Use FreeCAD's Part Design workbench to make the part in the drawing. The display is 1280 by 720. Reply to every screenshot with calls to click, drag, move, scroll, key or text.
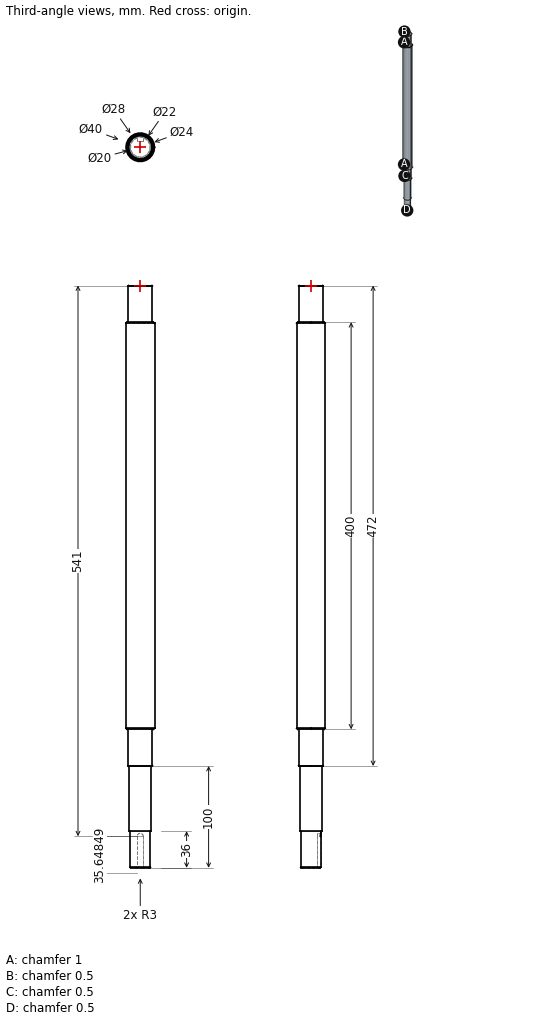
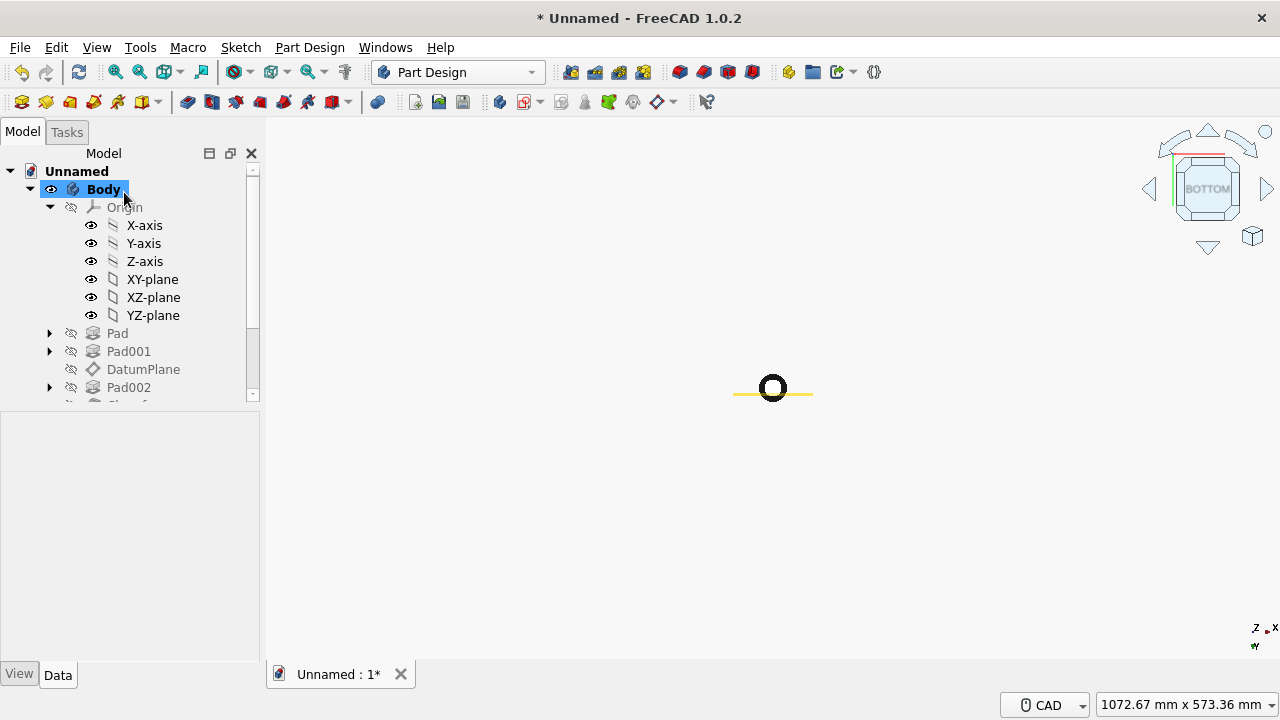
scroll(100, 275, down, 3)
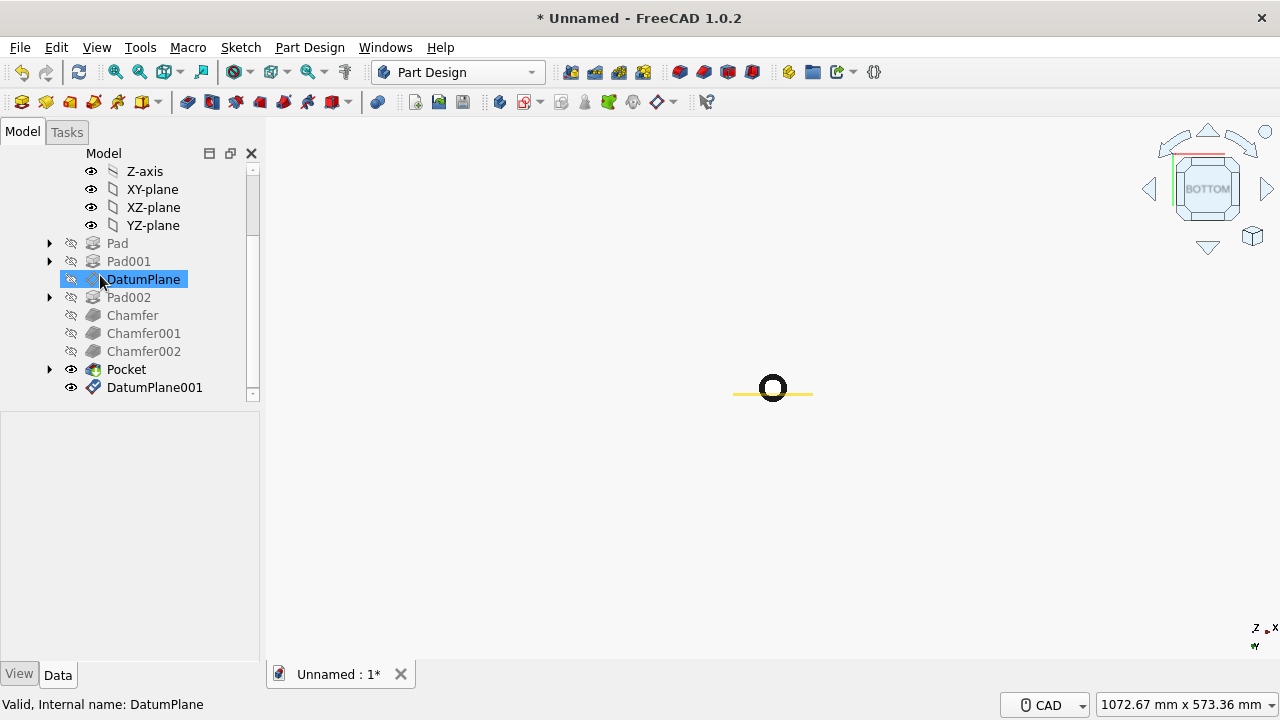
click(116, 387)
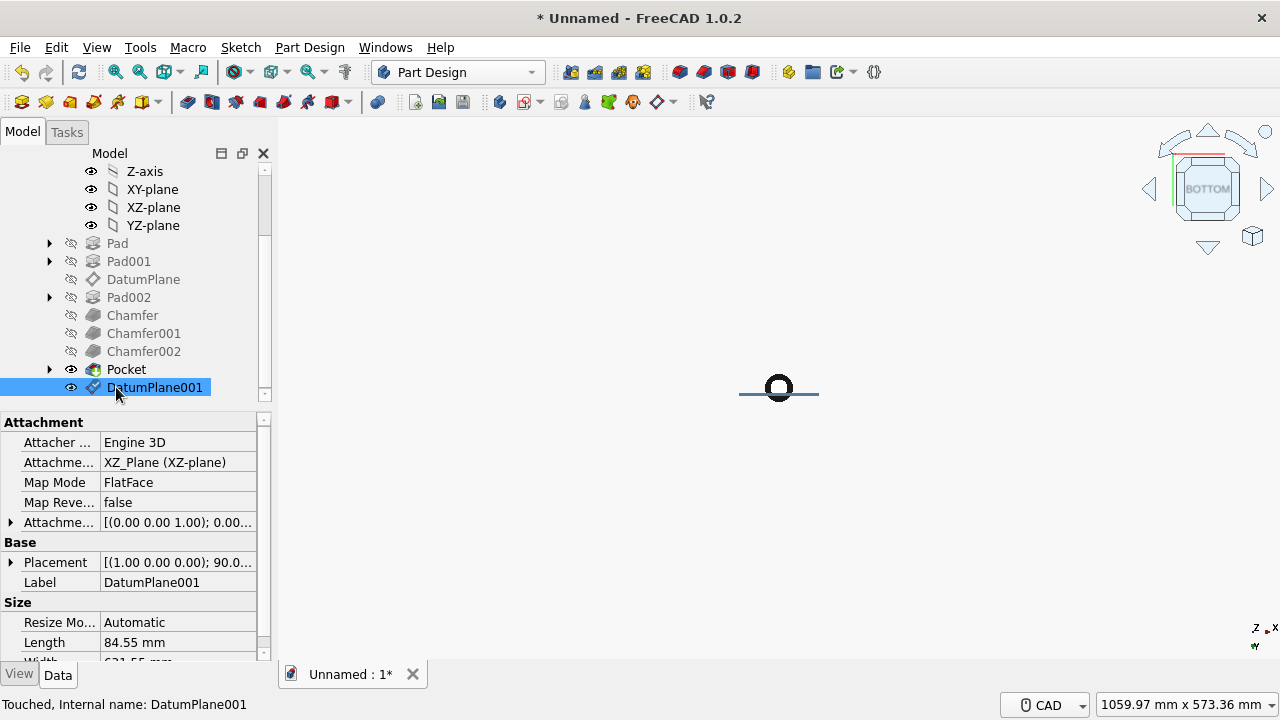
click(524, 102)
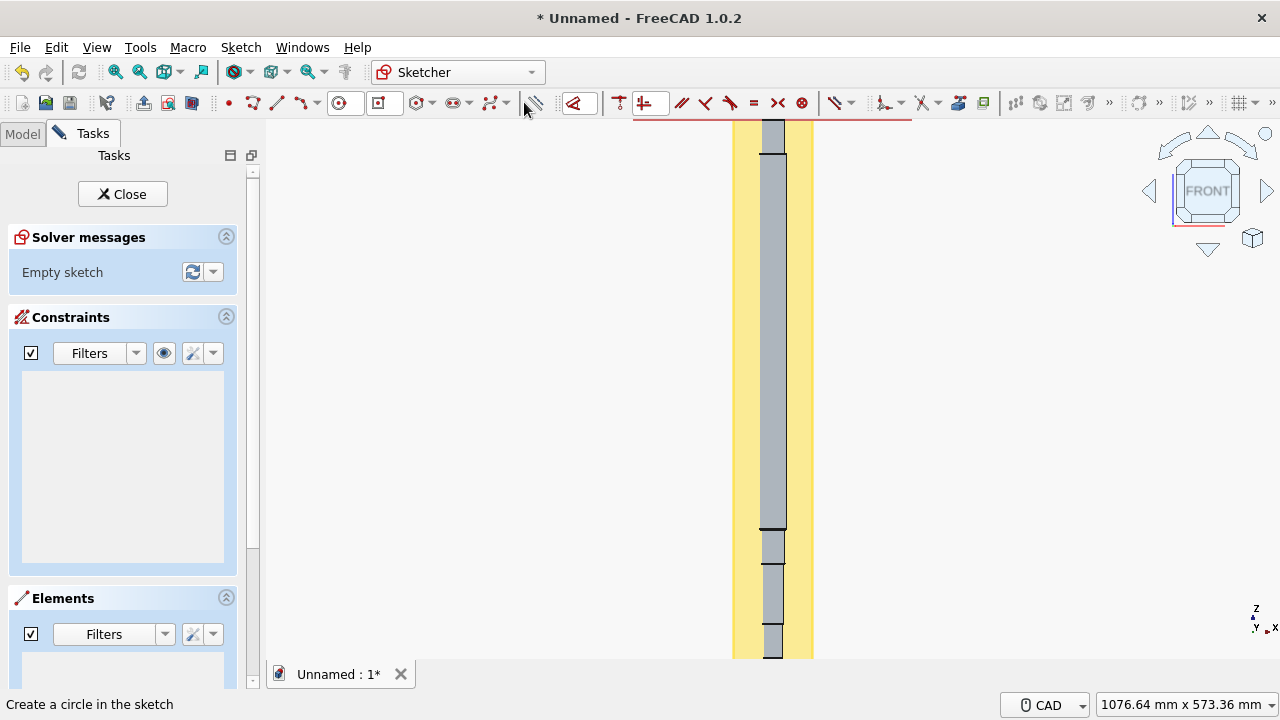
click(192, 104)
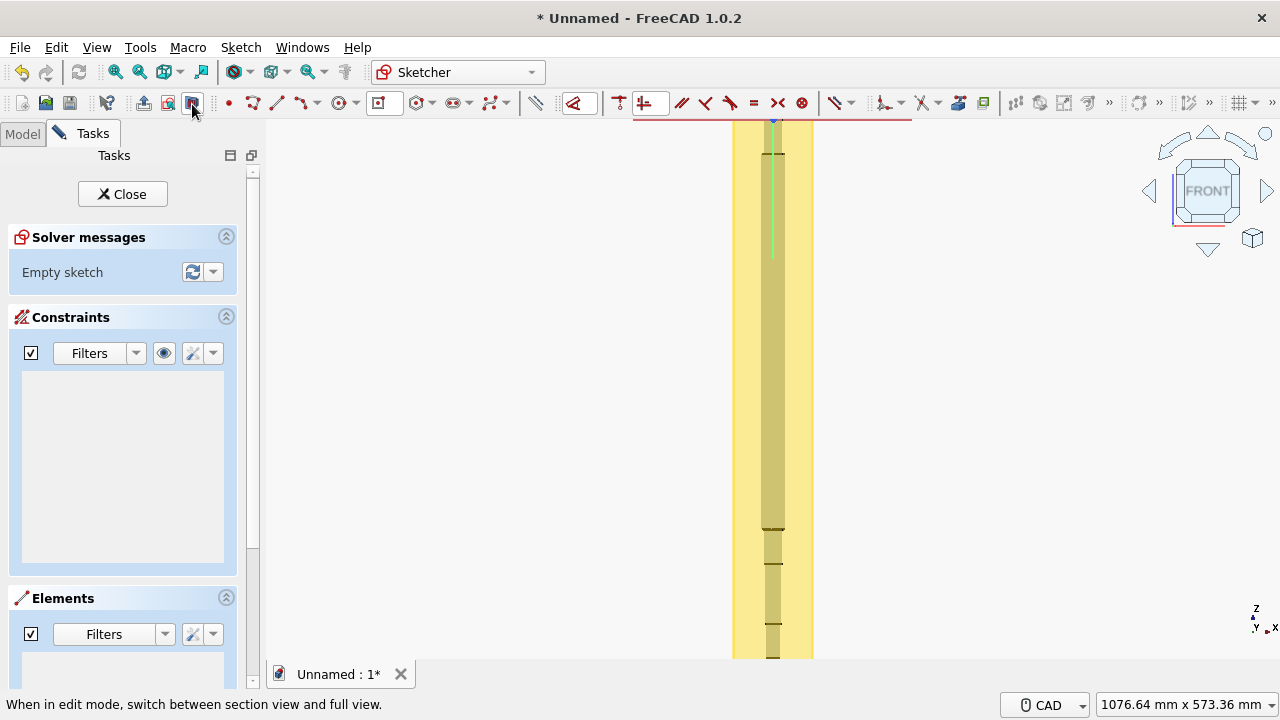
scroll(704, 389, down, 5)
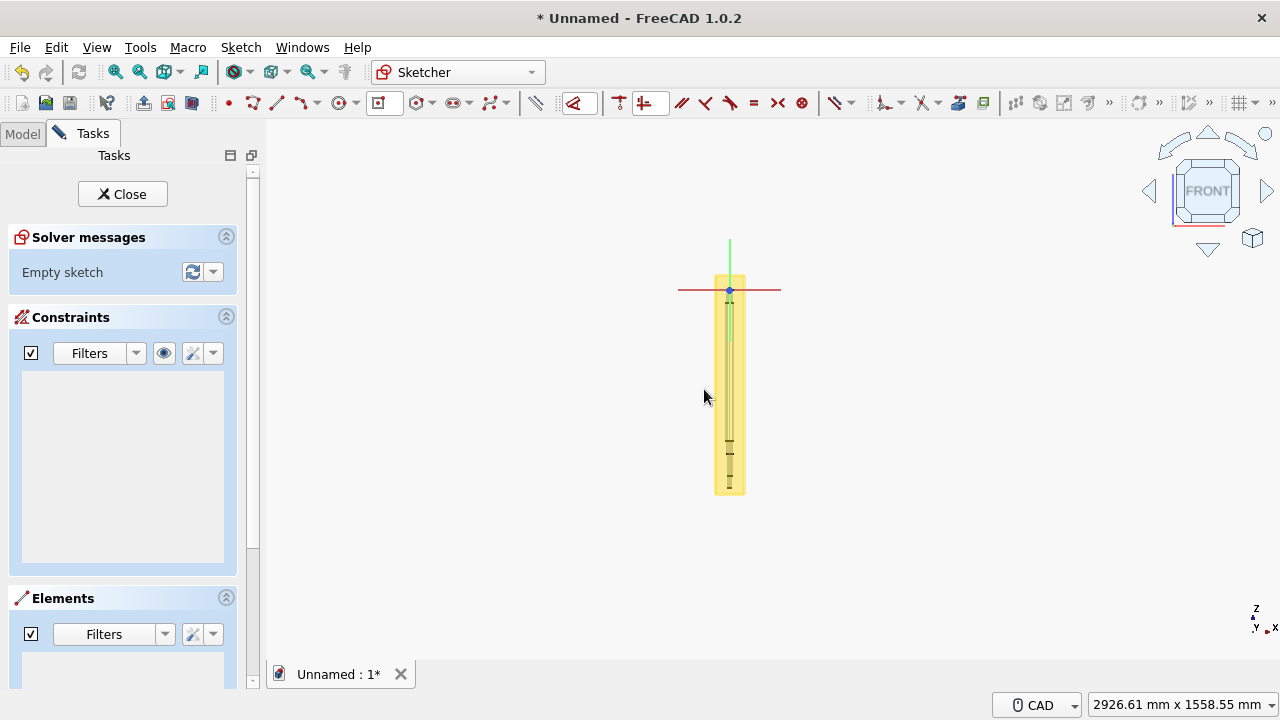
scroll(731, 489, up, 15)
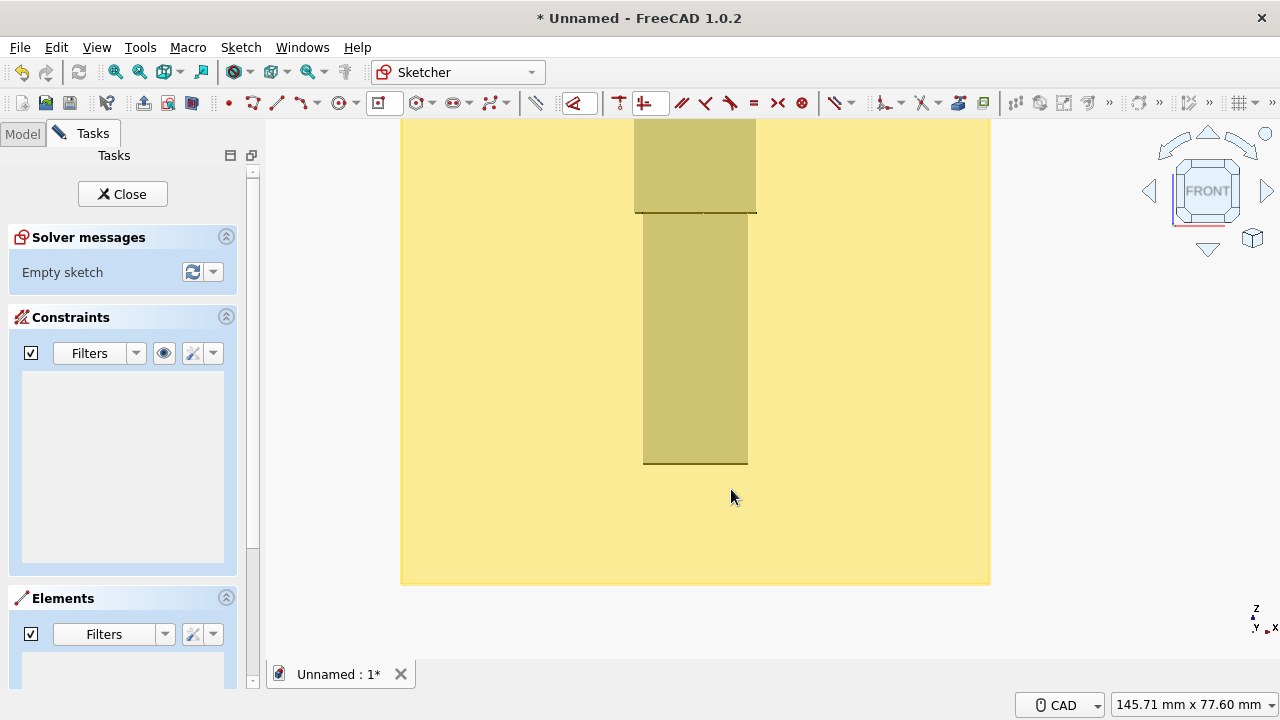
click(454, 104)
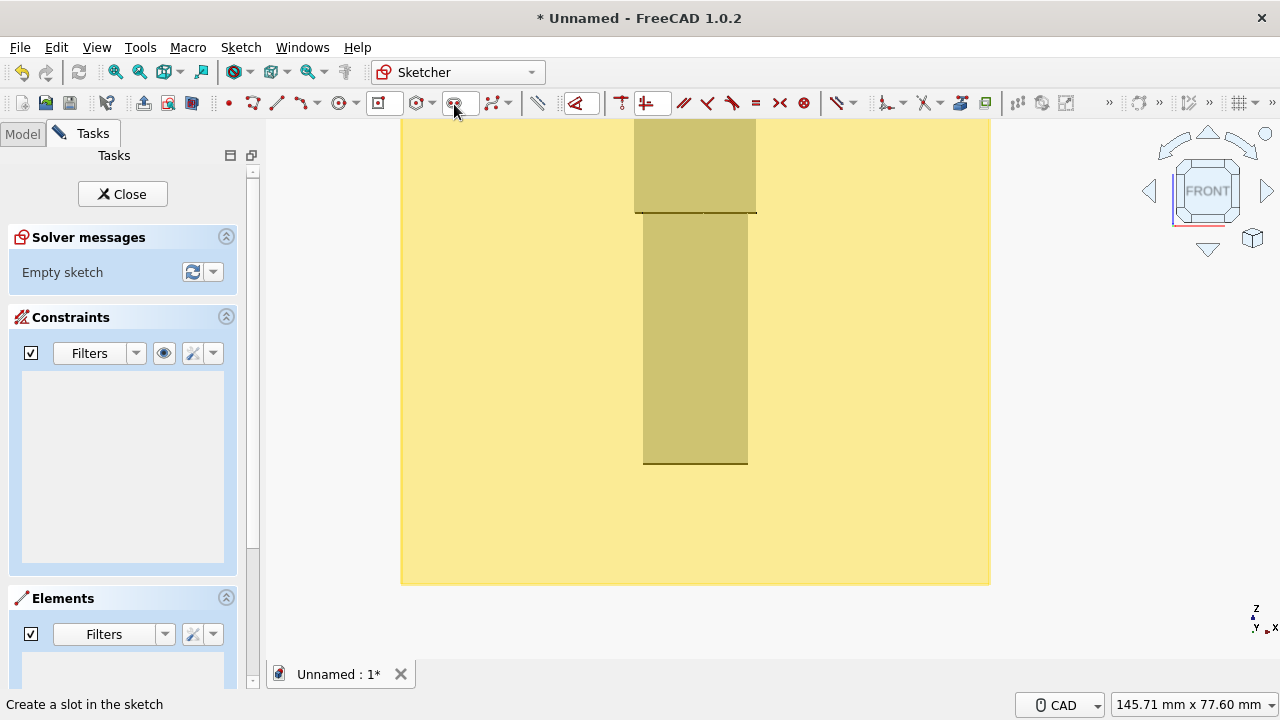
click(695, 496)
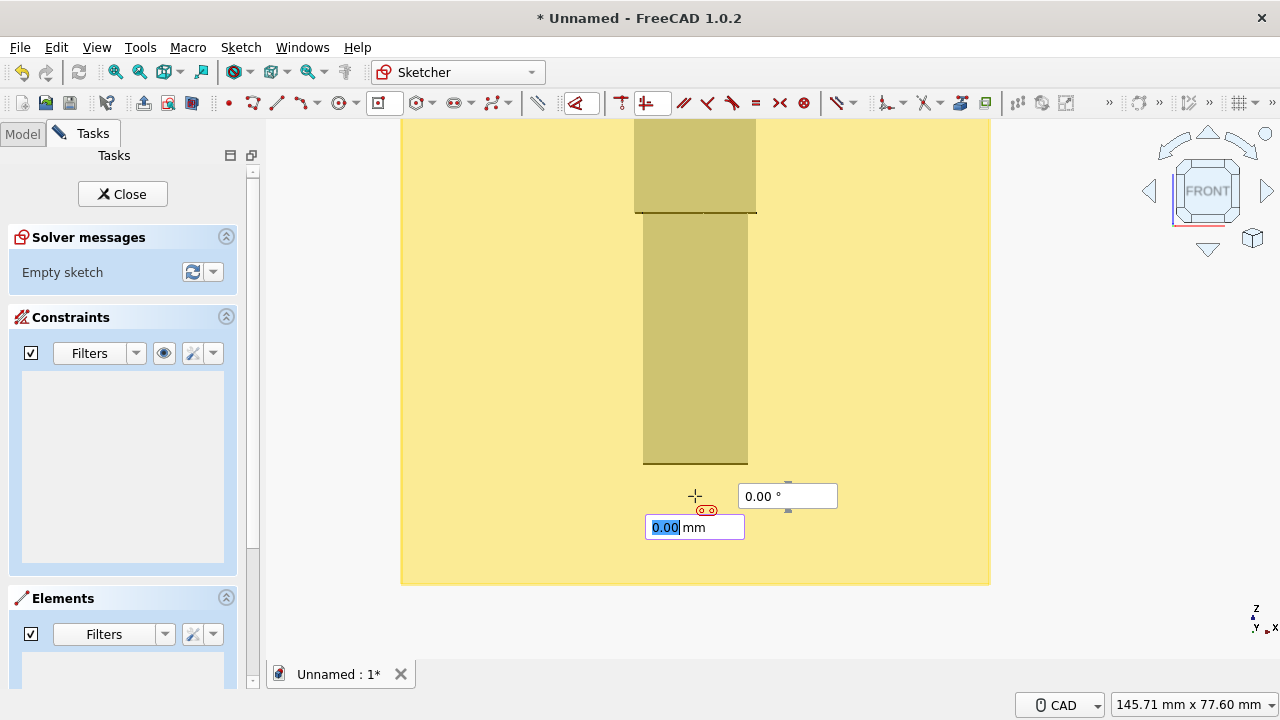
click(704, 248)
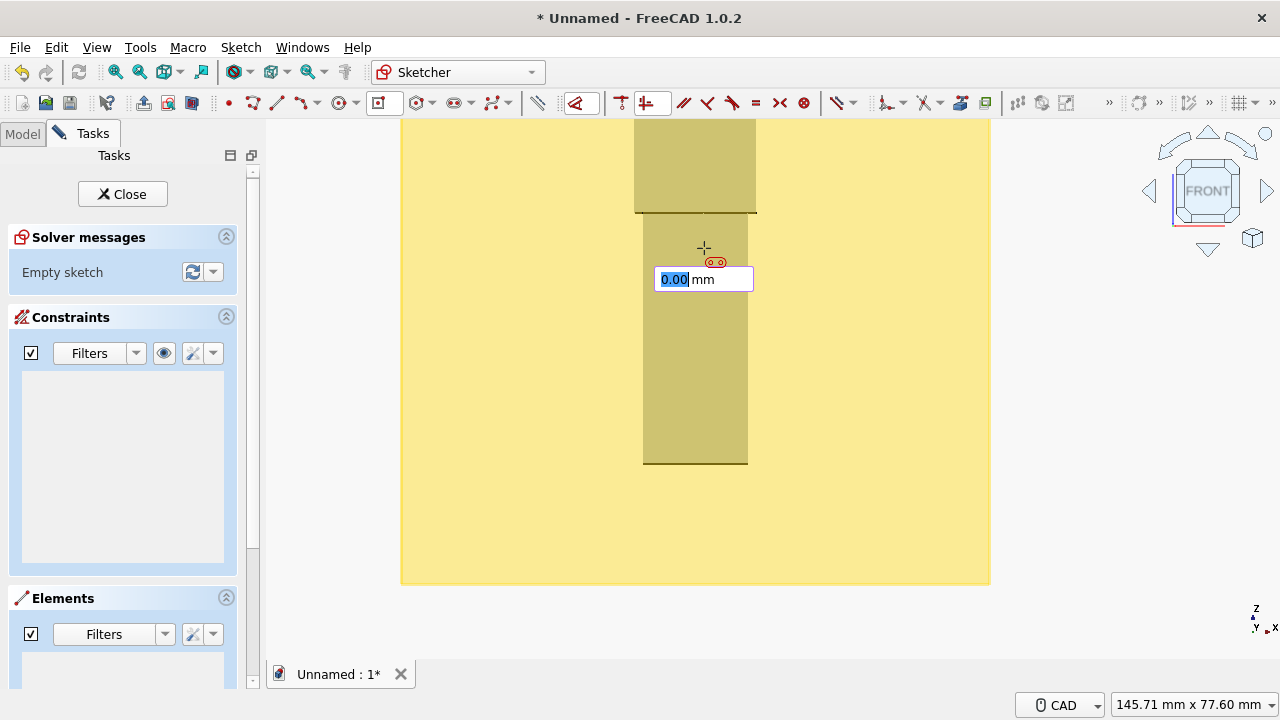
click(716, 372)
key(Escape)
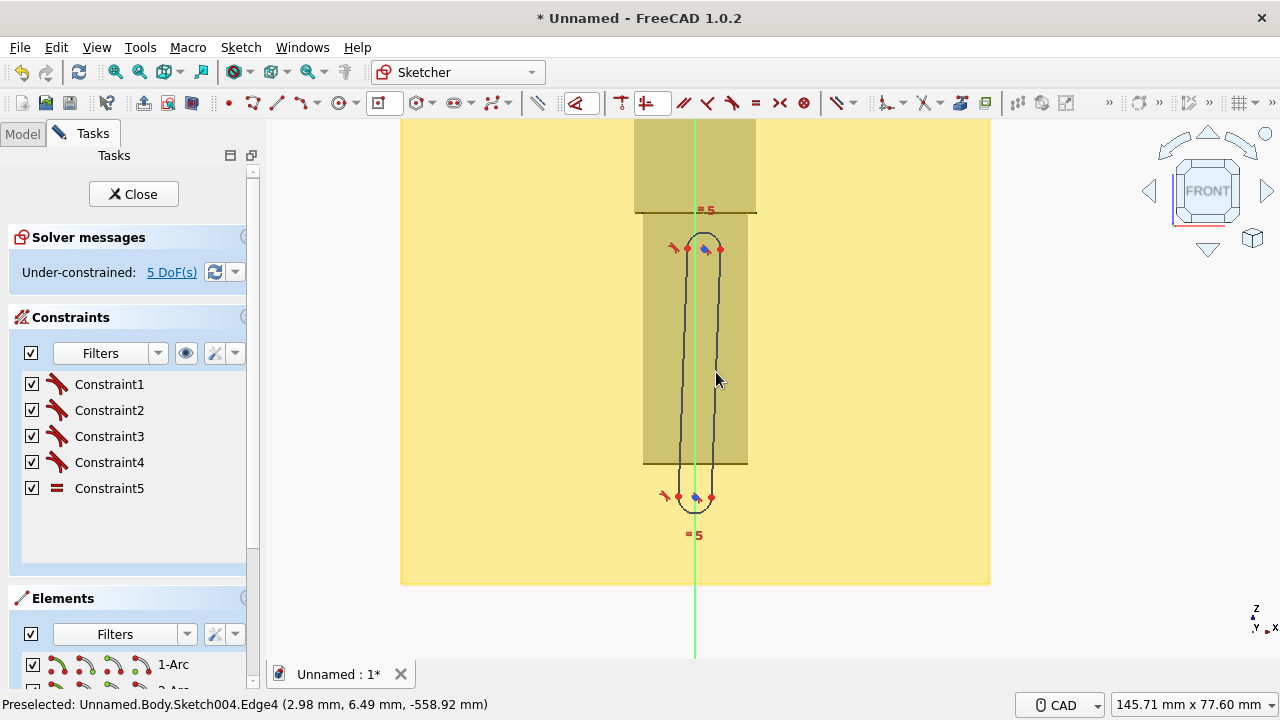
click(681, 422)